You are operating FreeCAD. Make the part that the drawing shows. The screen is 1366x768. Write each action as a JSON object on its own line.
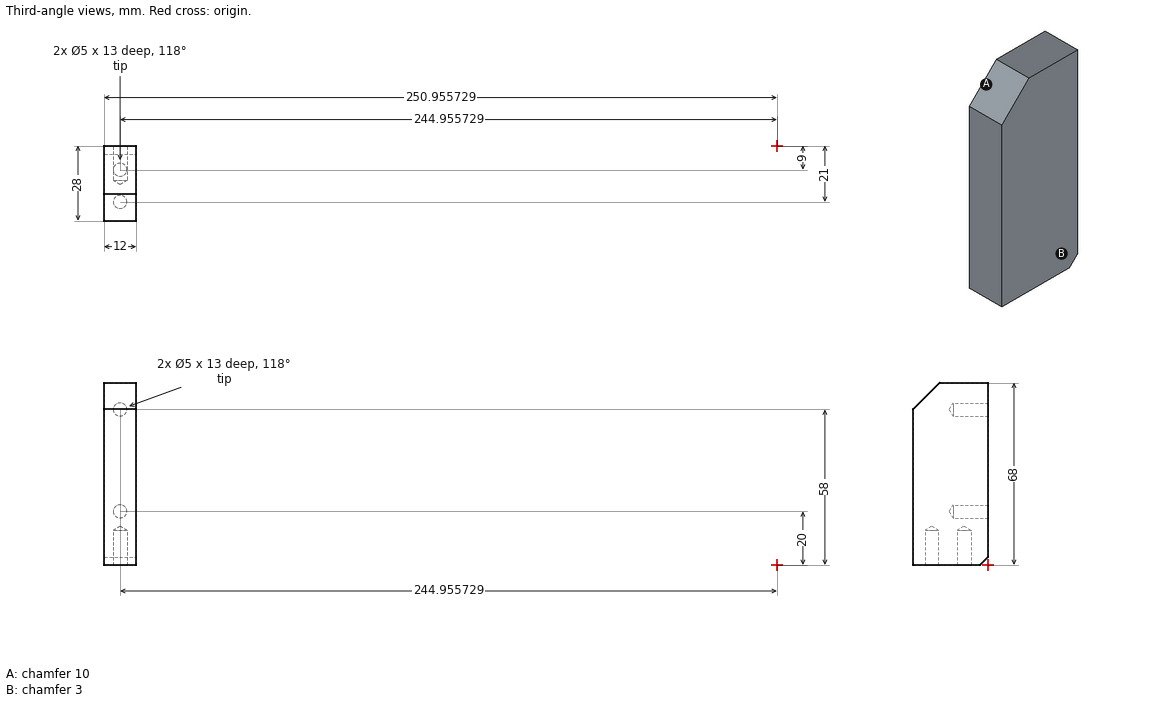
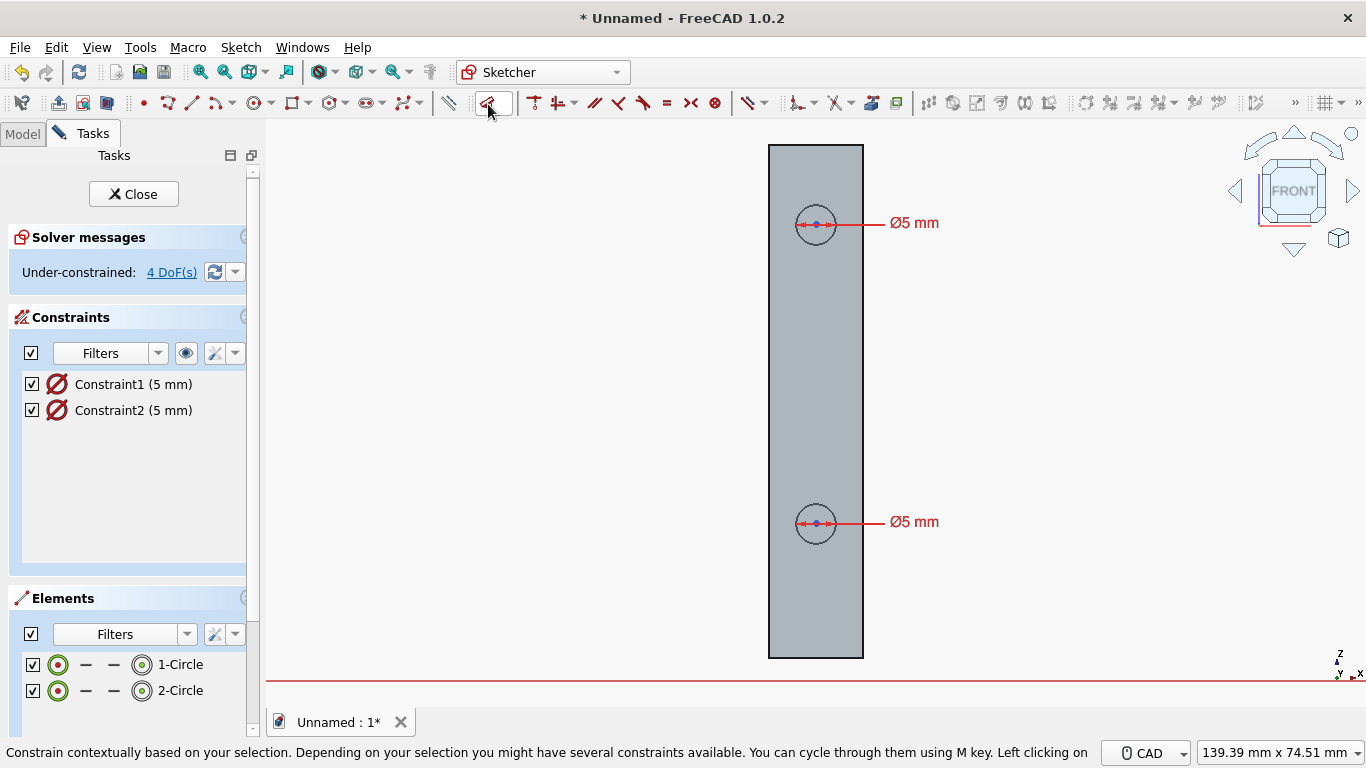
{"action": "left_click", "coordinate": [816, 225]}
{"action": "left_click", "coordinate": [782, 452]}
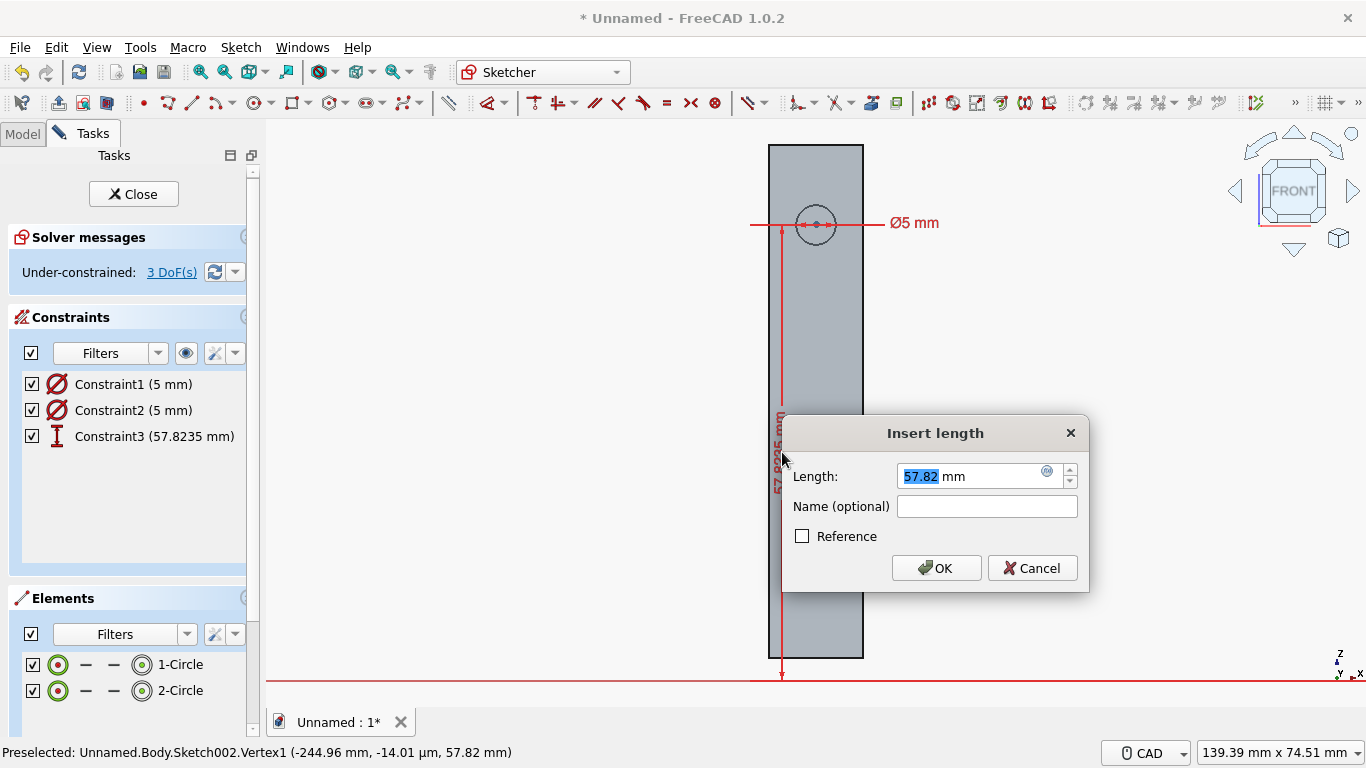
{"action": "type", "text": "58"}
{"action": "key", "text": "Return"}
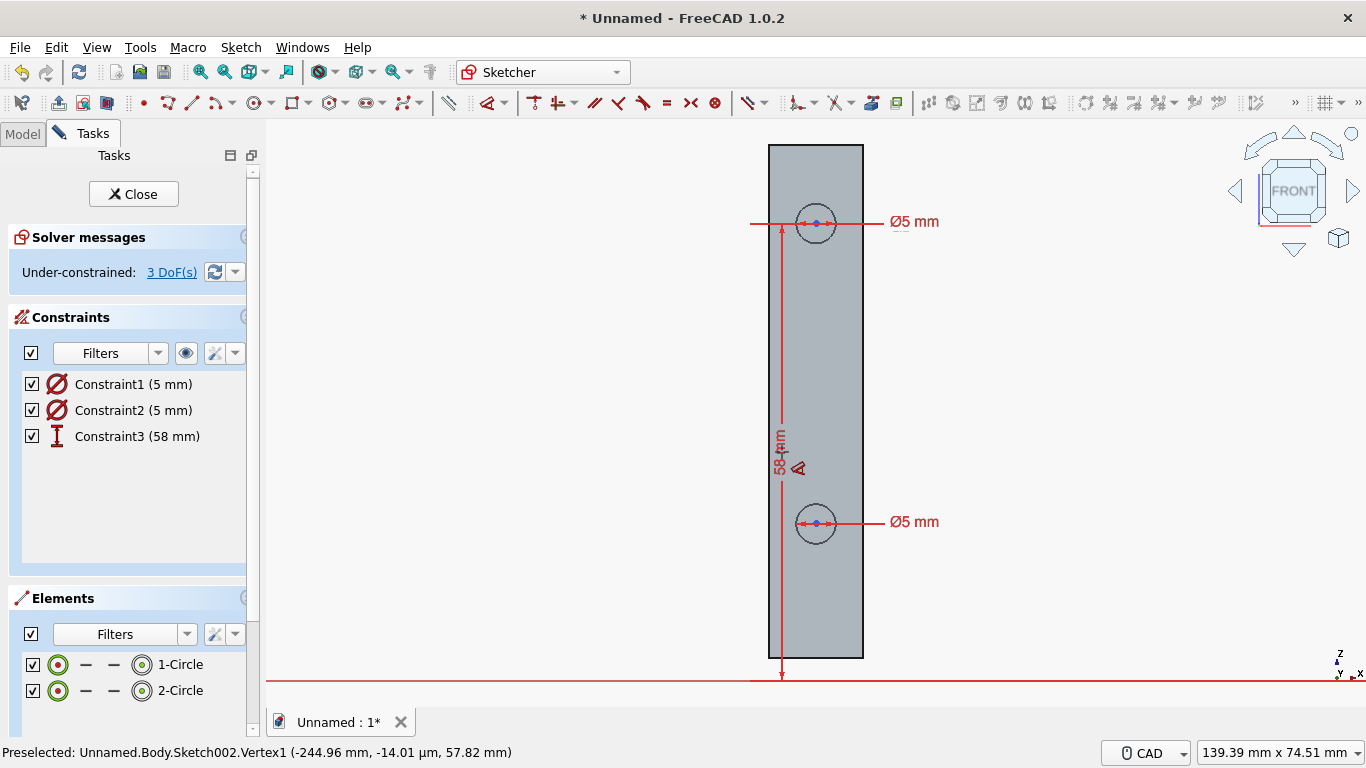
{"action": "left_click", "coordinate": [816, 524]}
{"action": "left_click", "coordinate": [782, 602]}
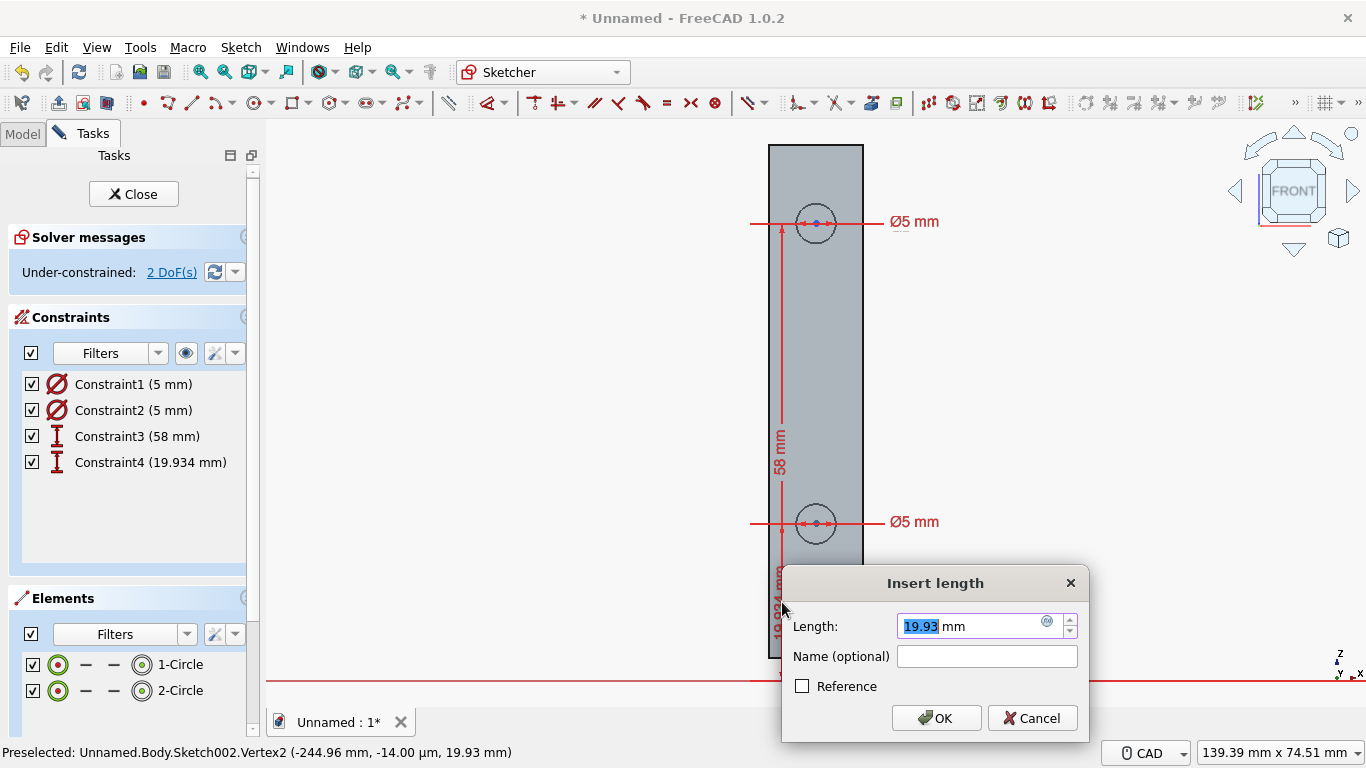
{"action": "type", "text": "20"}
{"action": "key", "text": "Return"}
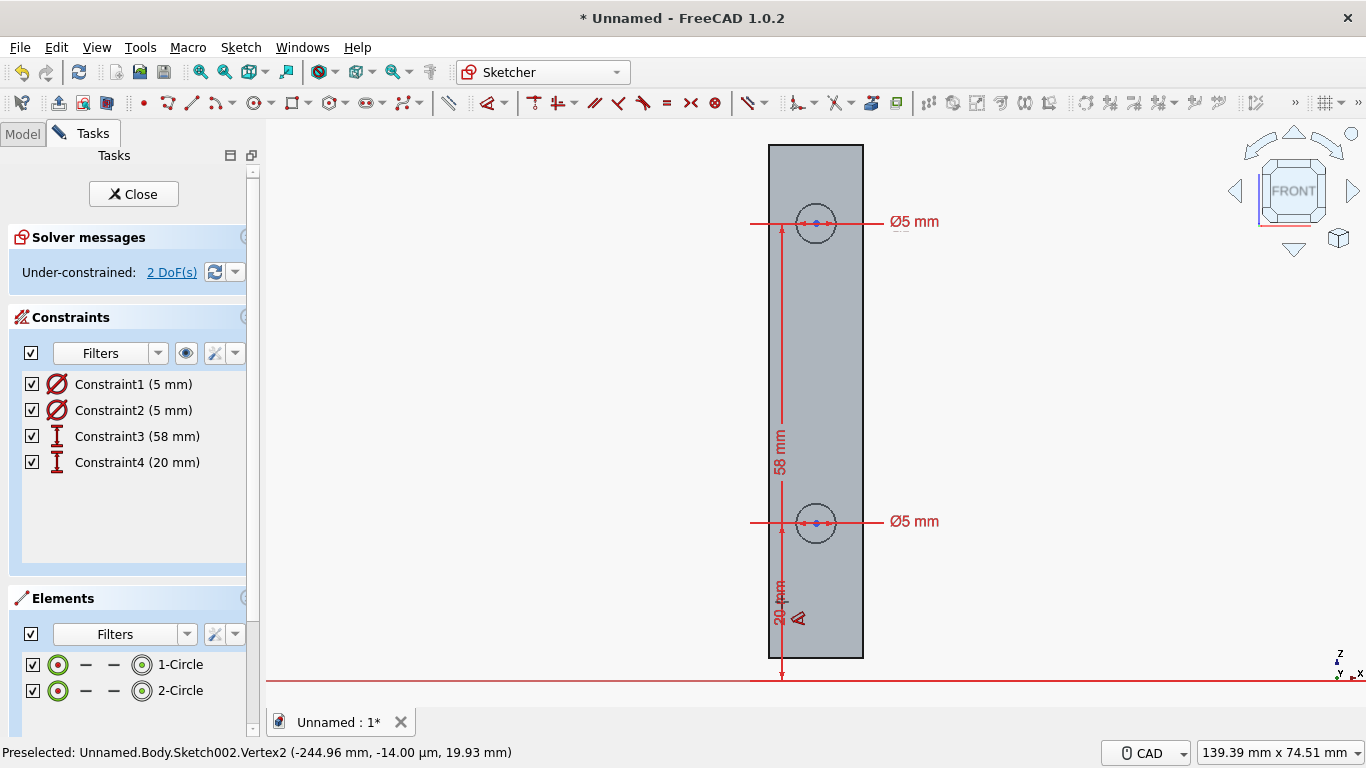
{"action": "left_click", "coordinate": [816, 224]}
{"action": "left_click", "coordinate": [1009, 190]}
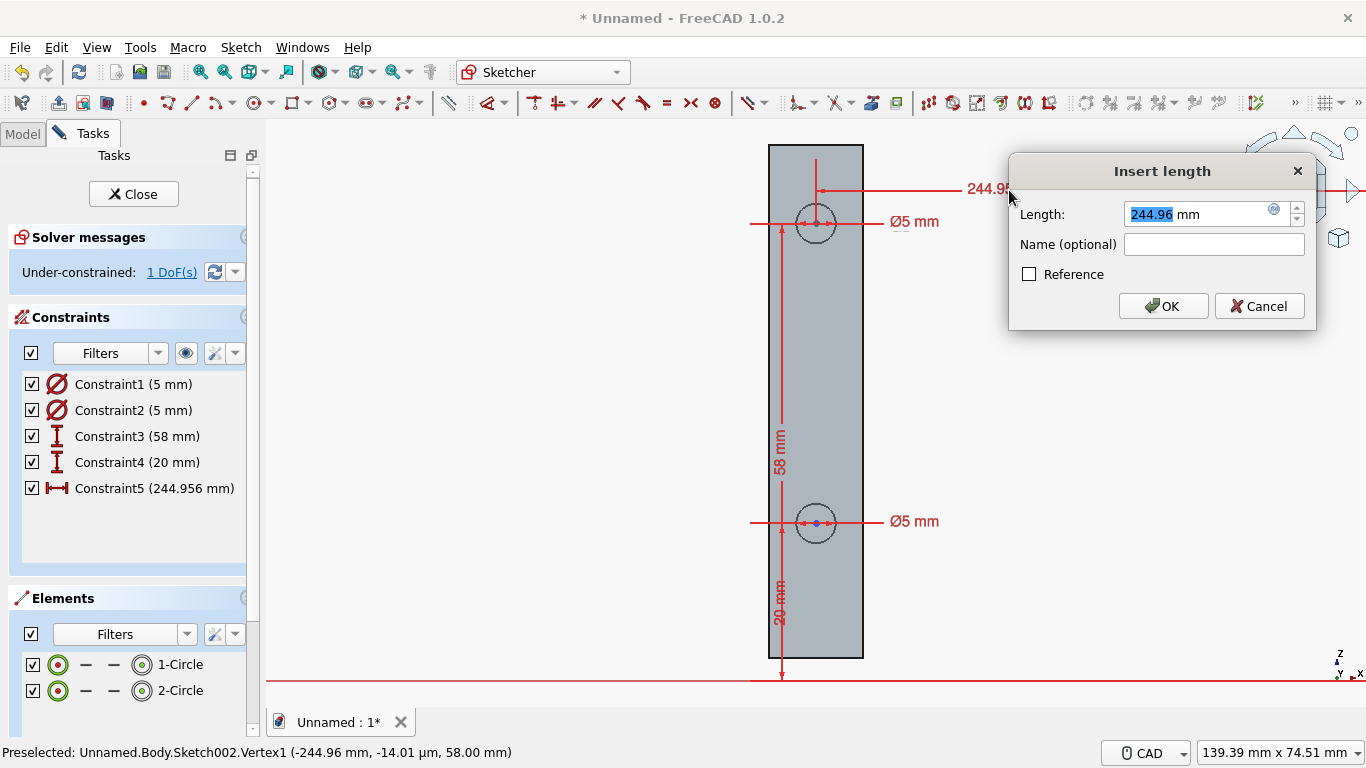
{"action": "type", "text": "244.955729"}
{"action": "key", "text": "Return"}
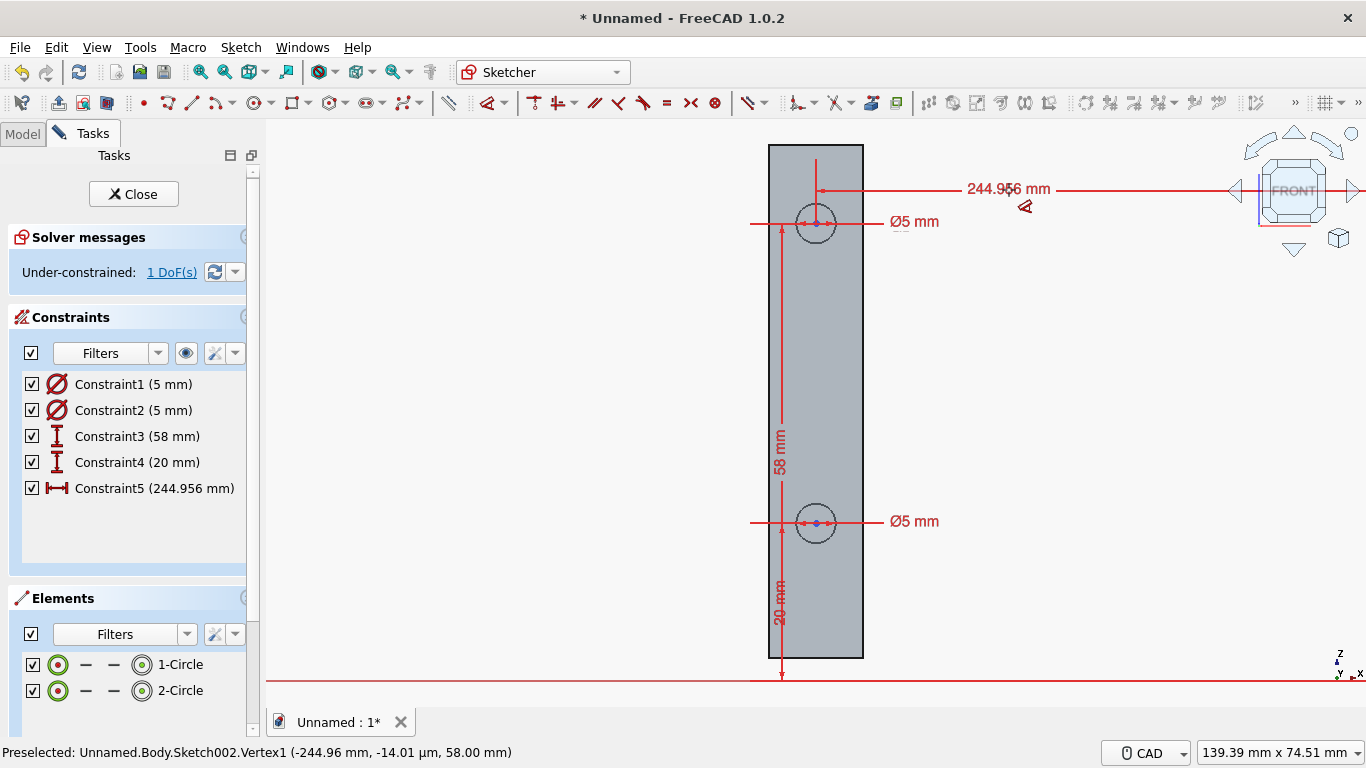
{"action": "left_click", "coordinate": [816, 523]}
{"action": "left_click", "coordinate": [1009, 489]}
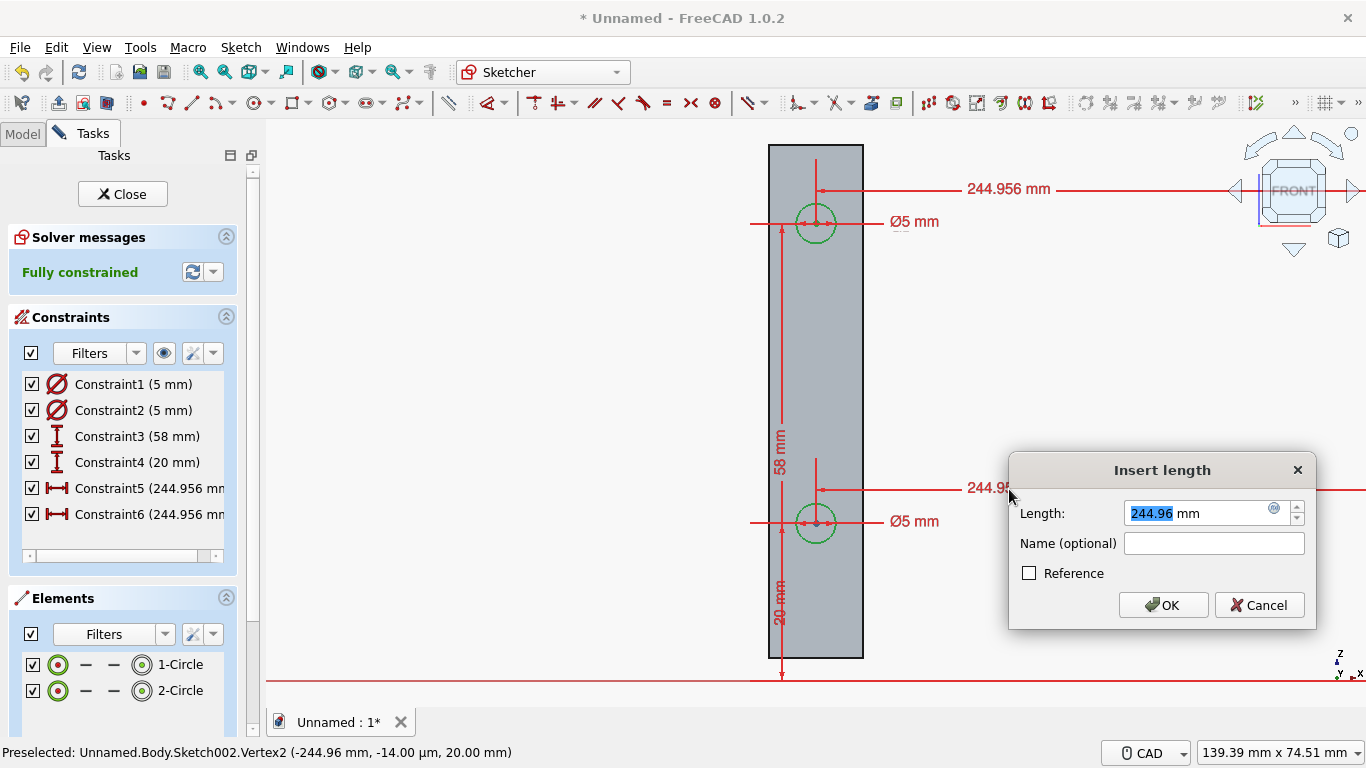
{"action": "type", "text": "244.955729"}
{"action": "key", "text": "Return"}
{"action": "key", "text": "Escape"}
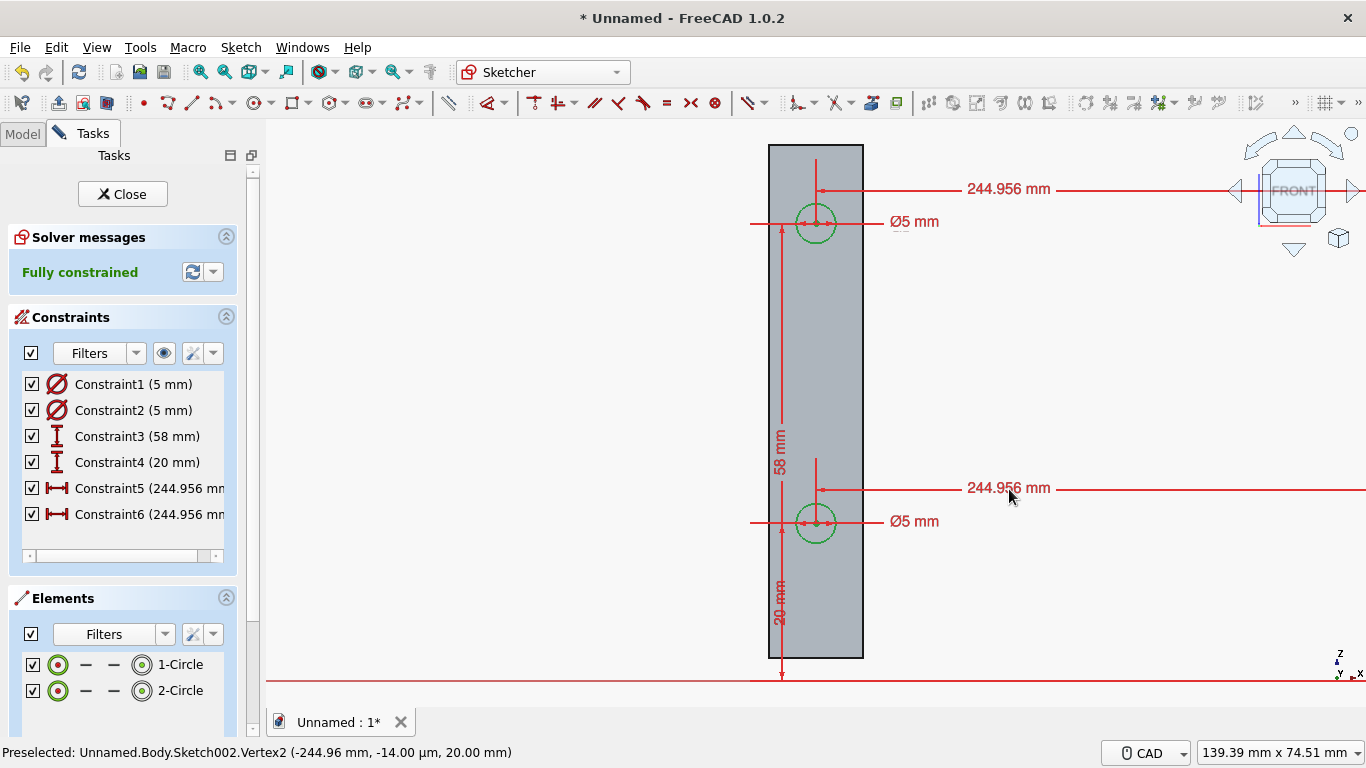
{"action": "left_click", "coordinate": [123, 194]}